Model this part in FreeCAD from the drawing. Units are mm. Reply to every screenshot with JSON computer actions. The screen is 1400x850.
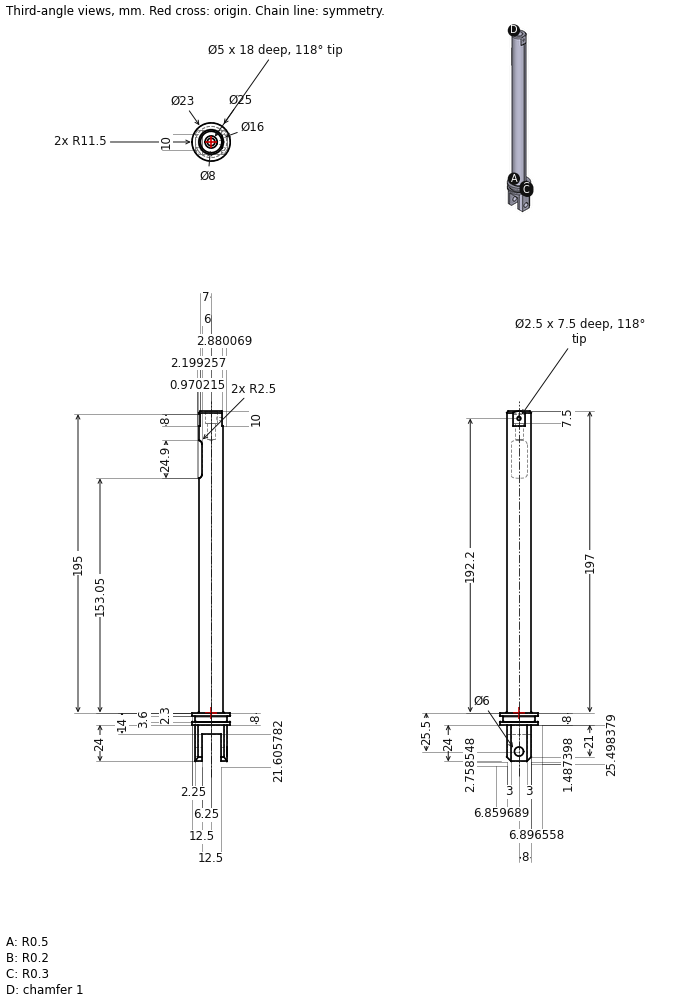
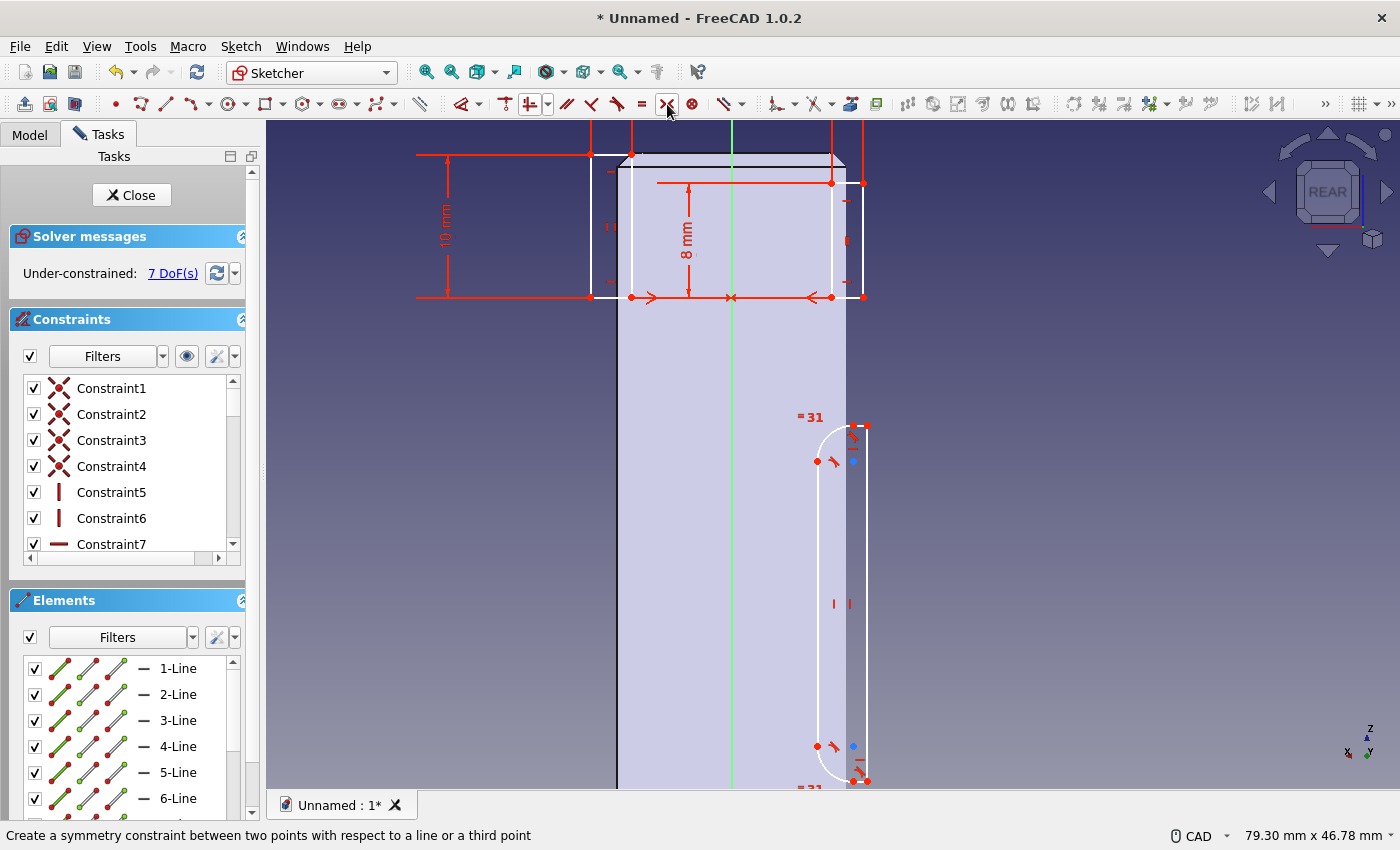
{"action": "left_click", "coordinate": [460, 104]}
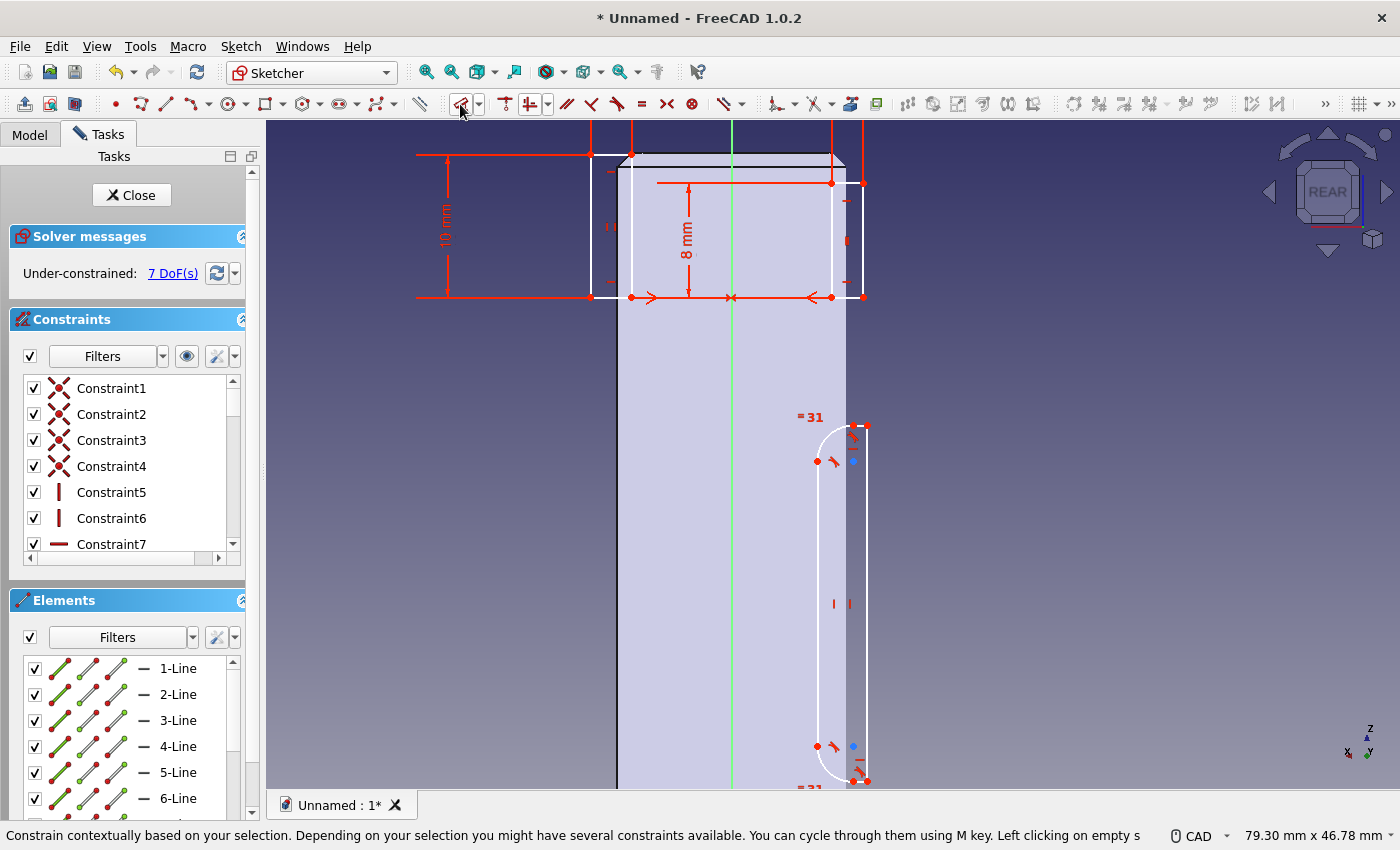
{"action": "left_click", "coordinate": [837, 430]}
{"action": "left_click", "coordinate": [822, 402]}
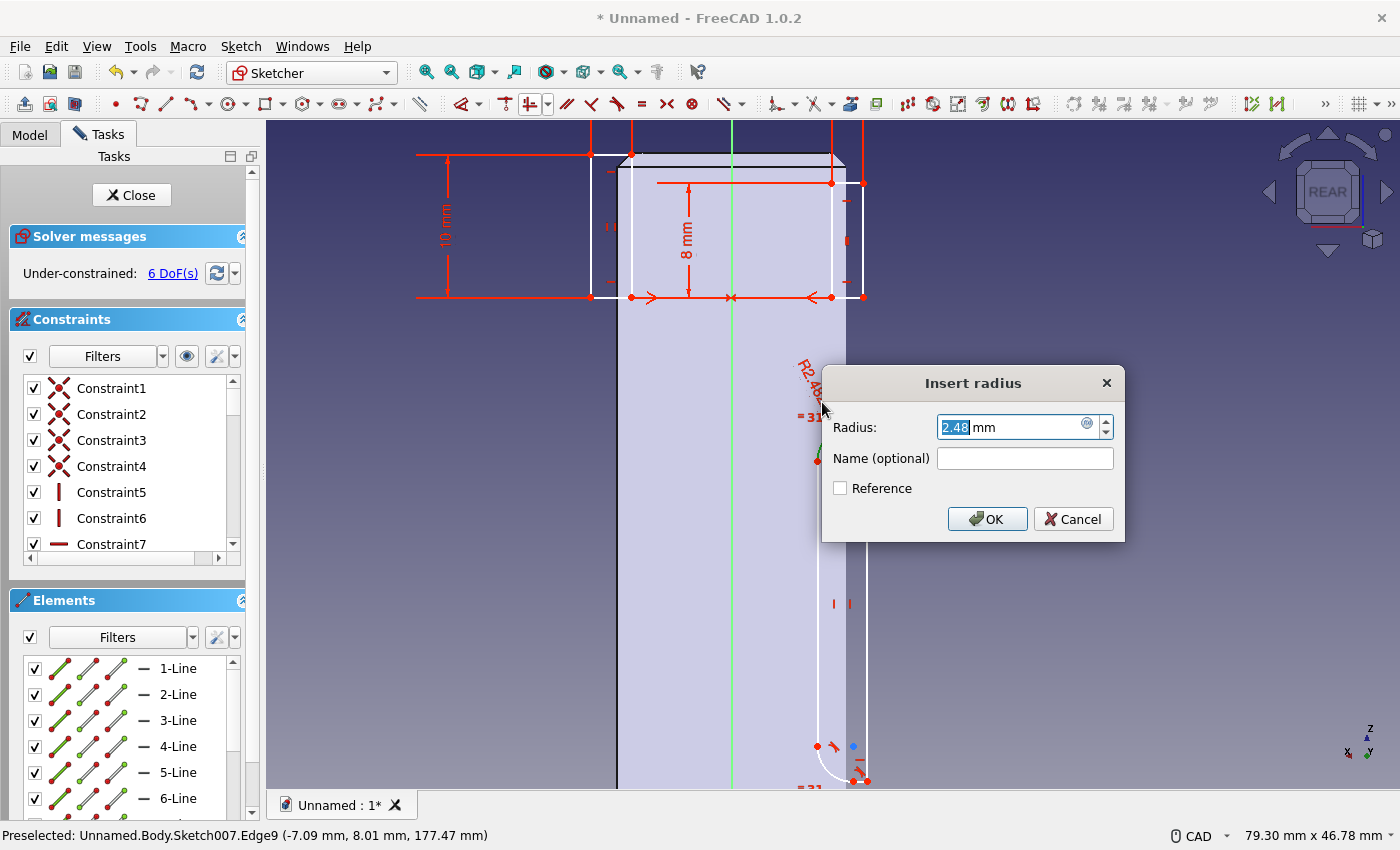
{"action": "type", "text": "2.5"}
{"action": "key", "text": "Return"}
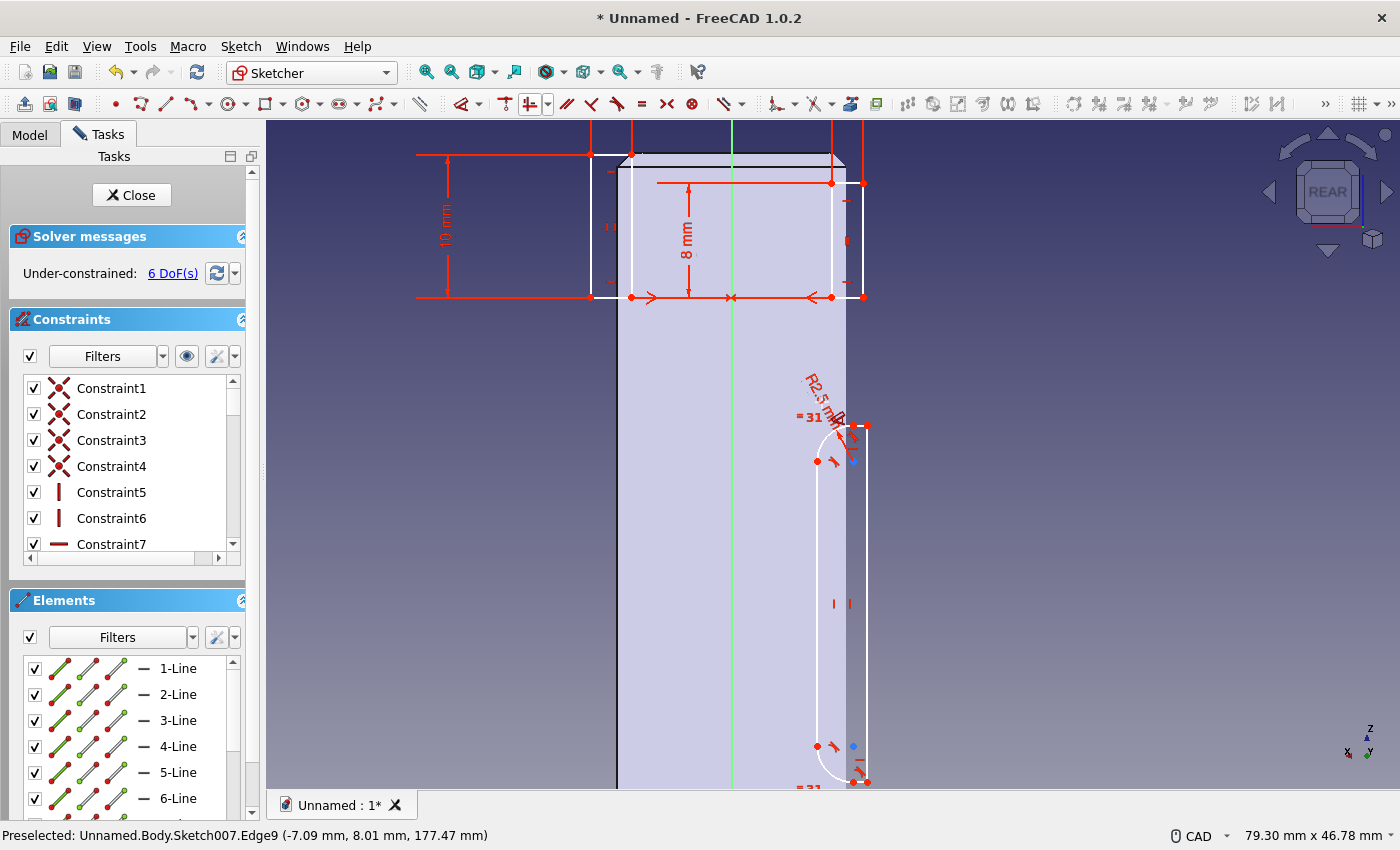
{"action": "left_click", "coordinate": [832, 183]}
{"action": "left_click", "coordinate": [782, 149]}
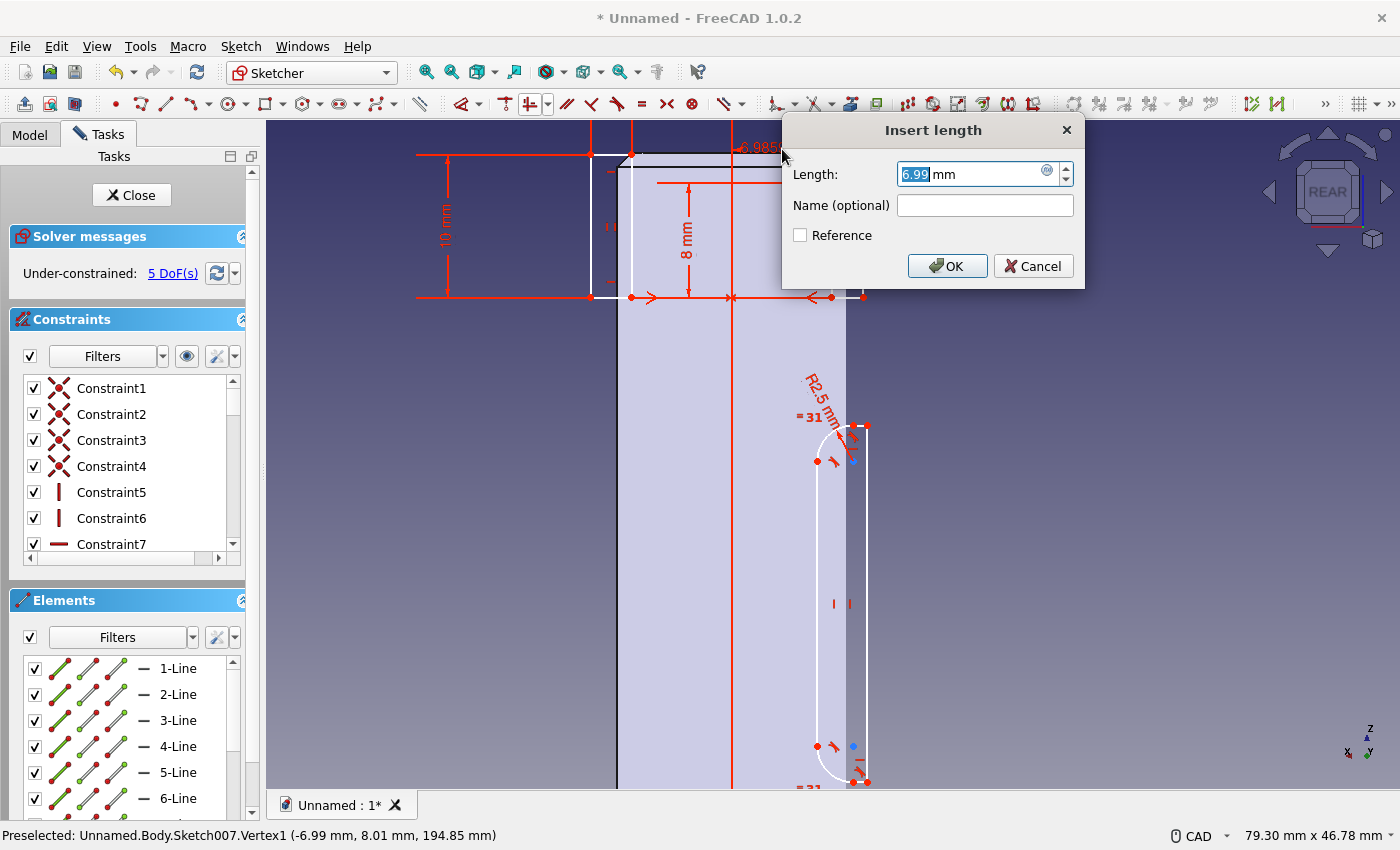
{"action": "type", "text": "7"}
{"action": "key", "text": "Return"}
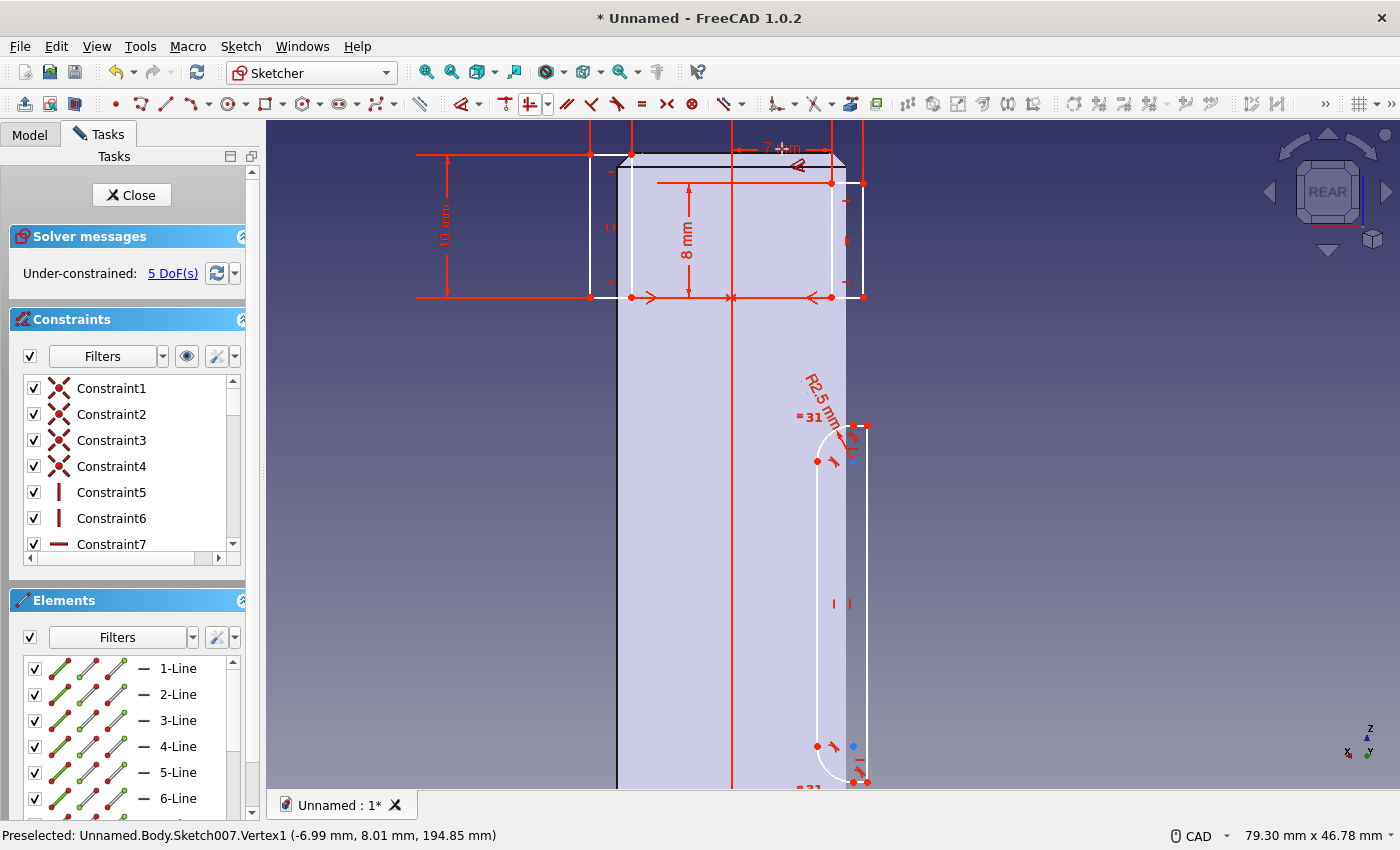
{"action": "left_click", "coordinate": [817, 461]}
{"action": "left_click", "coordinate": [775, 427]}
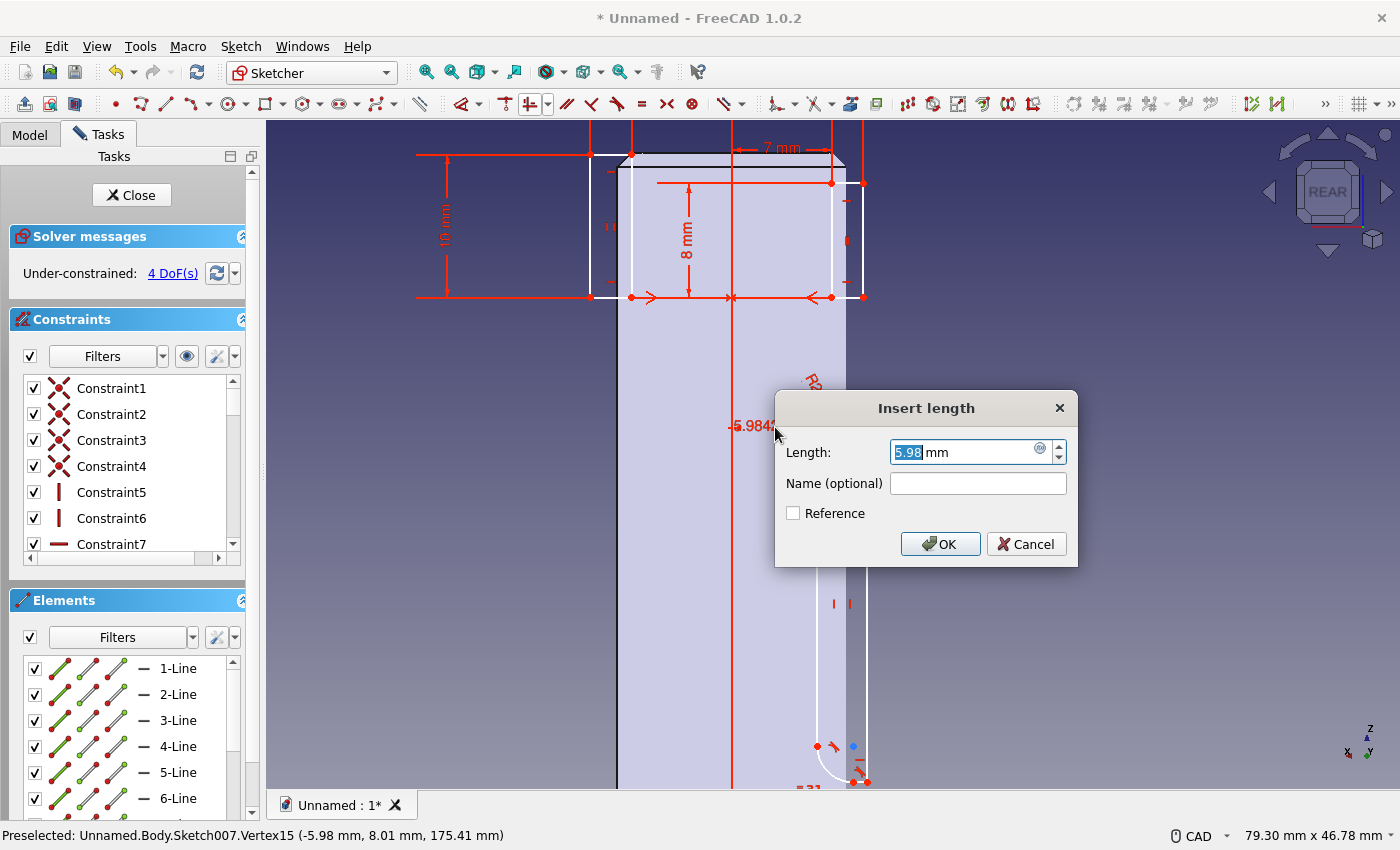
{"action": "type", "text": "6"}
{"action": "key", "text": "Return"}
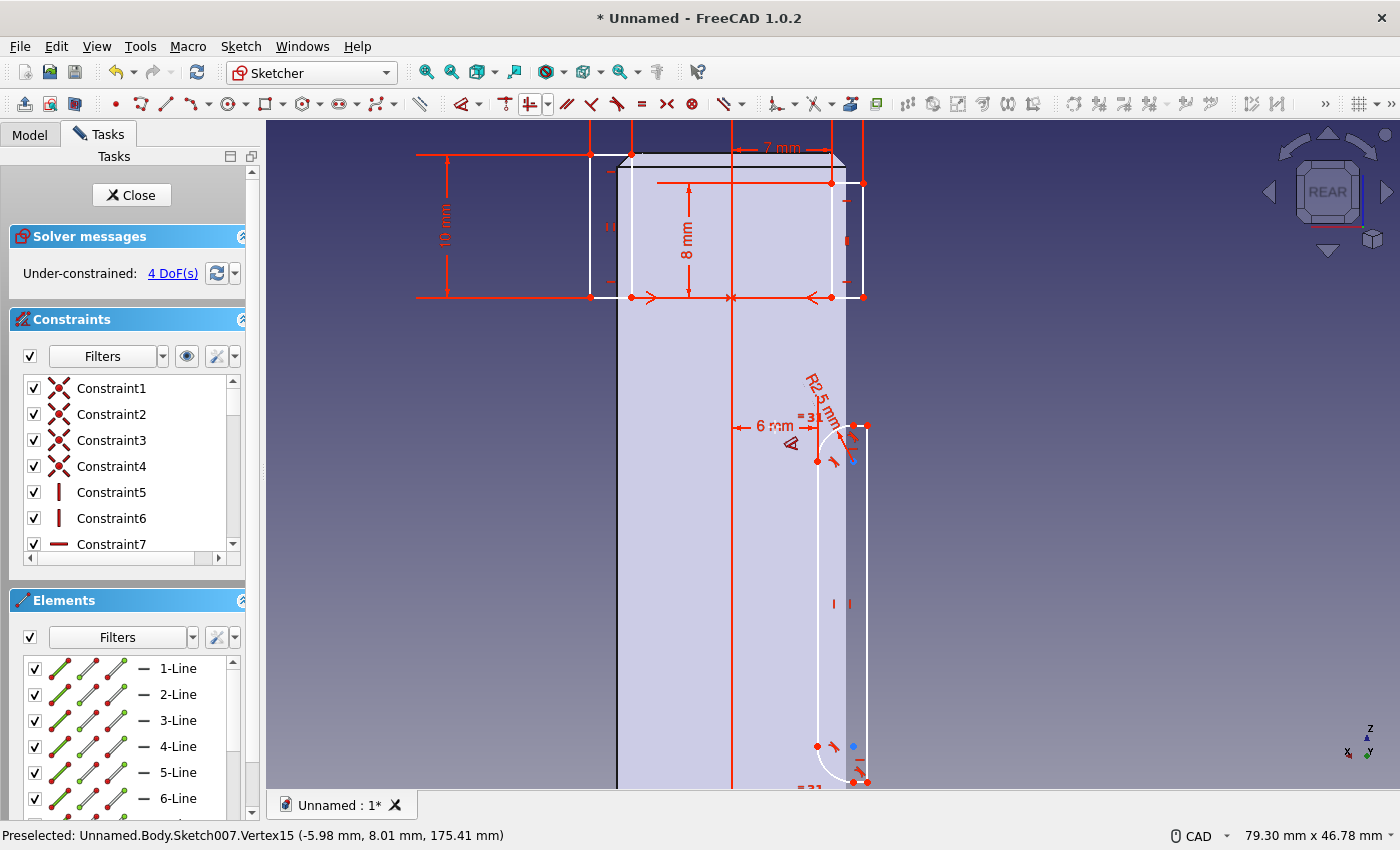
{"action": "left_click", "coordinate": [867, 675]}
{"action": "left_click", "coordinate": [901, 593]}